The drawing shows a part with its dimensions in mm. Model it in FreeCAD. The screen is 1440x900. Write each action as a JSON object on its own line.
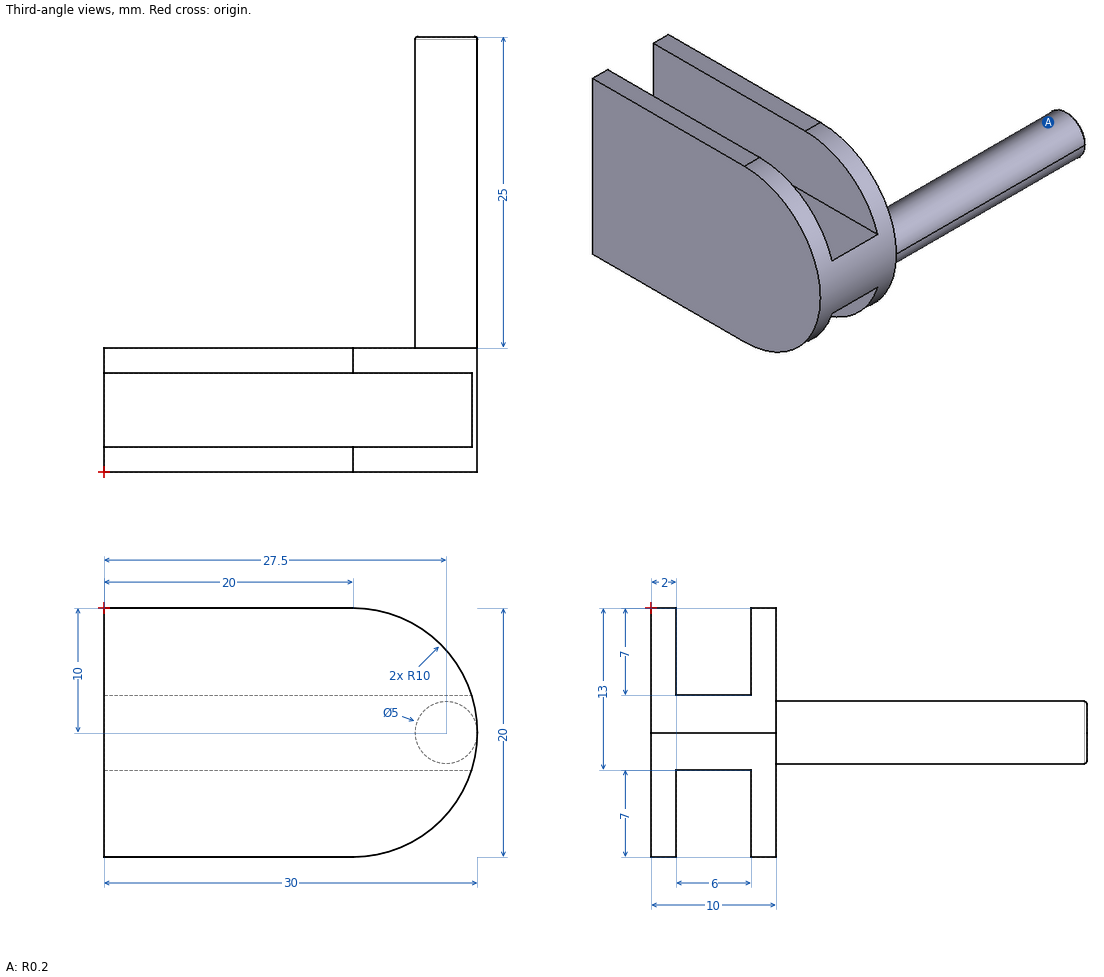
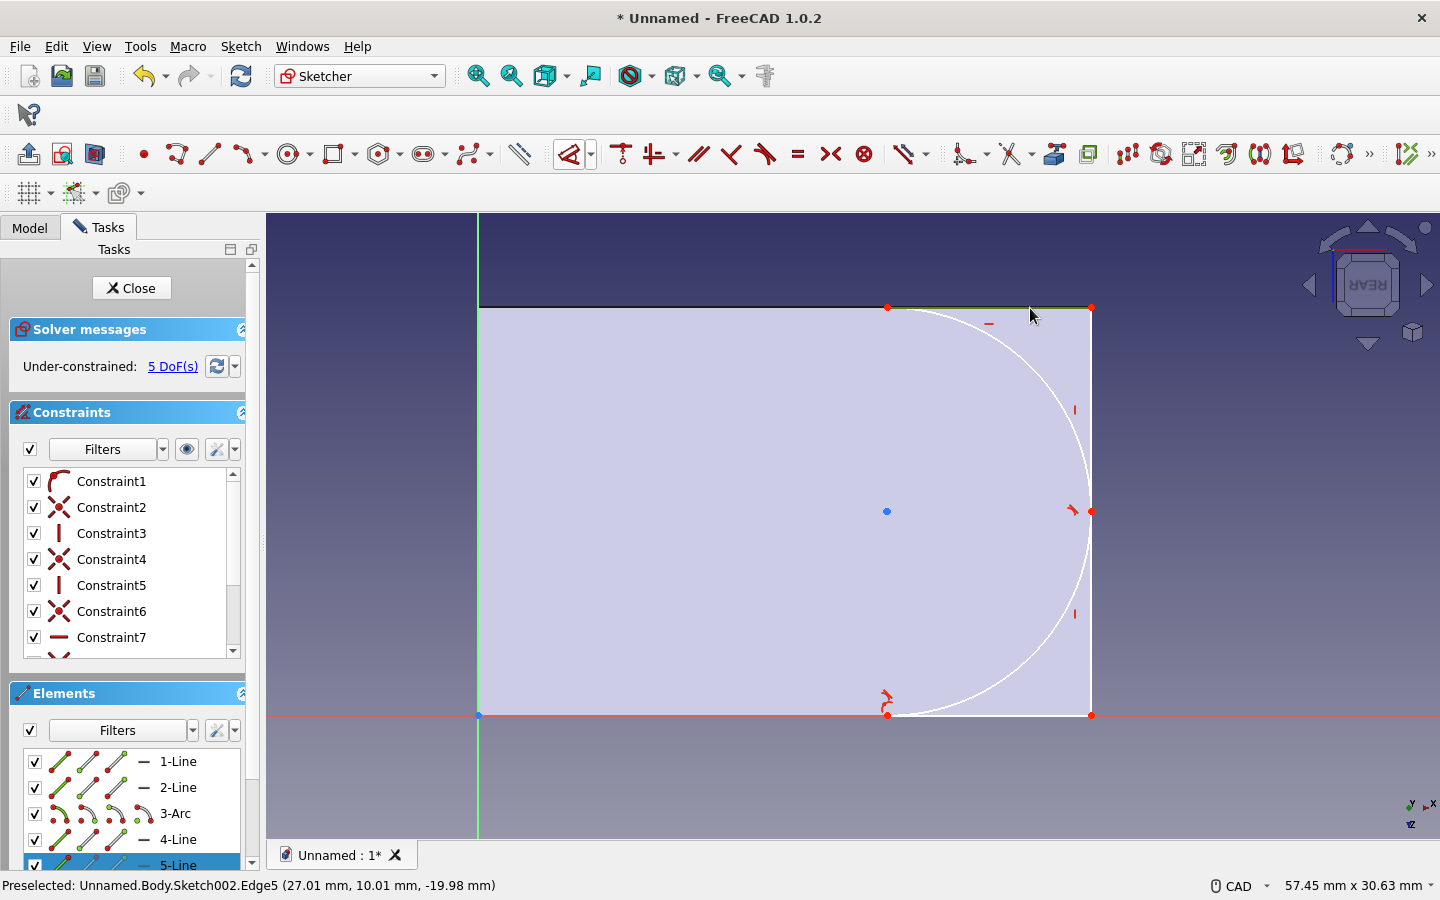
{"action": "left_click", "coordinate": [1069, 419]}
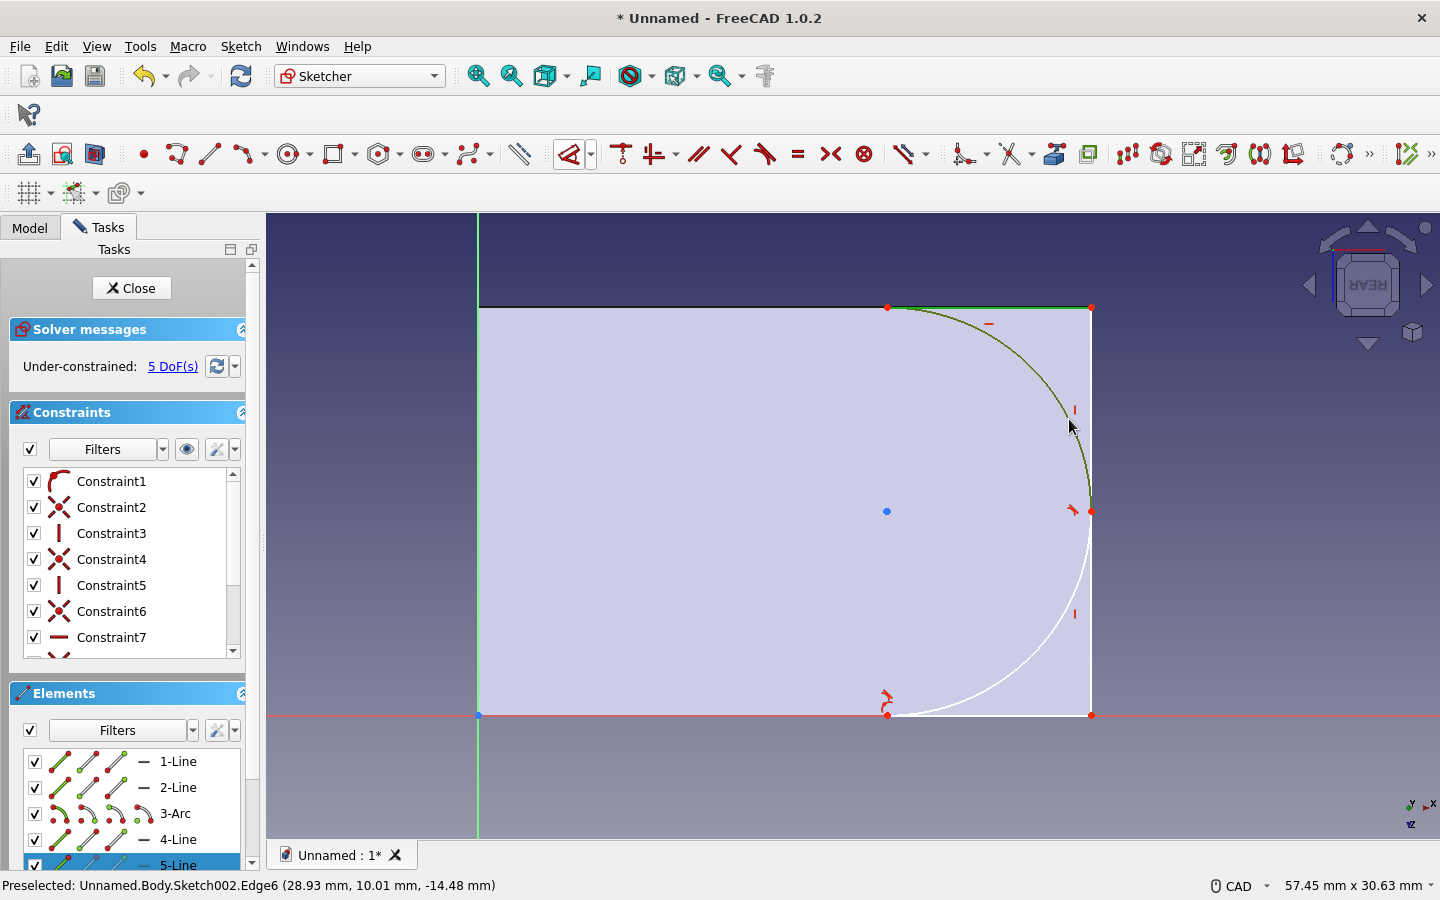
{"action": "left_click", "coordinate": [765, 154]}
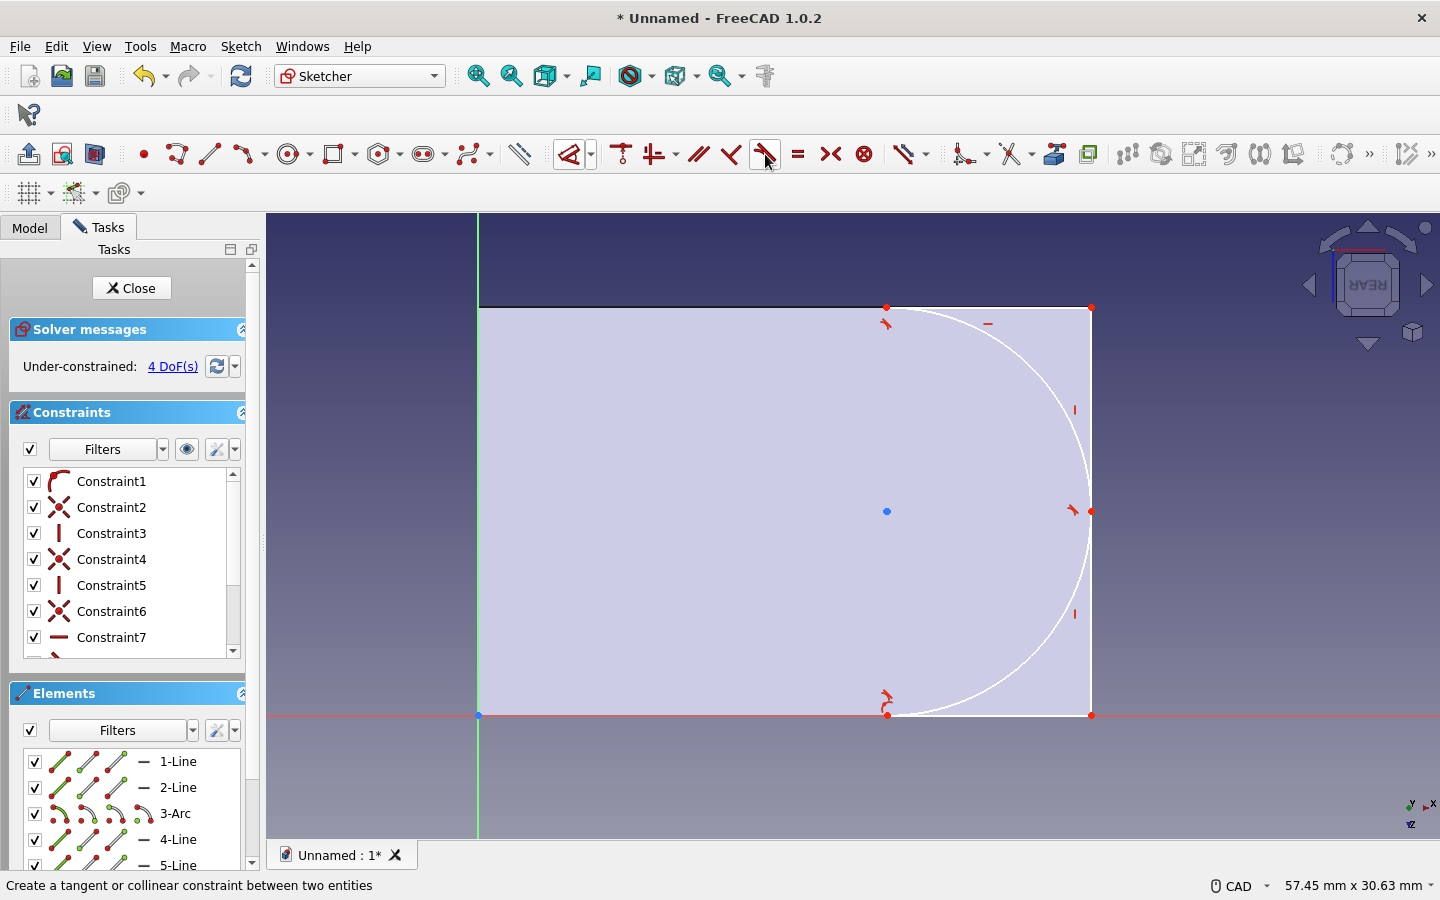
{"action": "left_click", "coordinate": [1030, 716]}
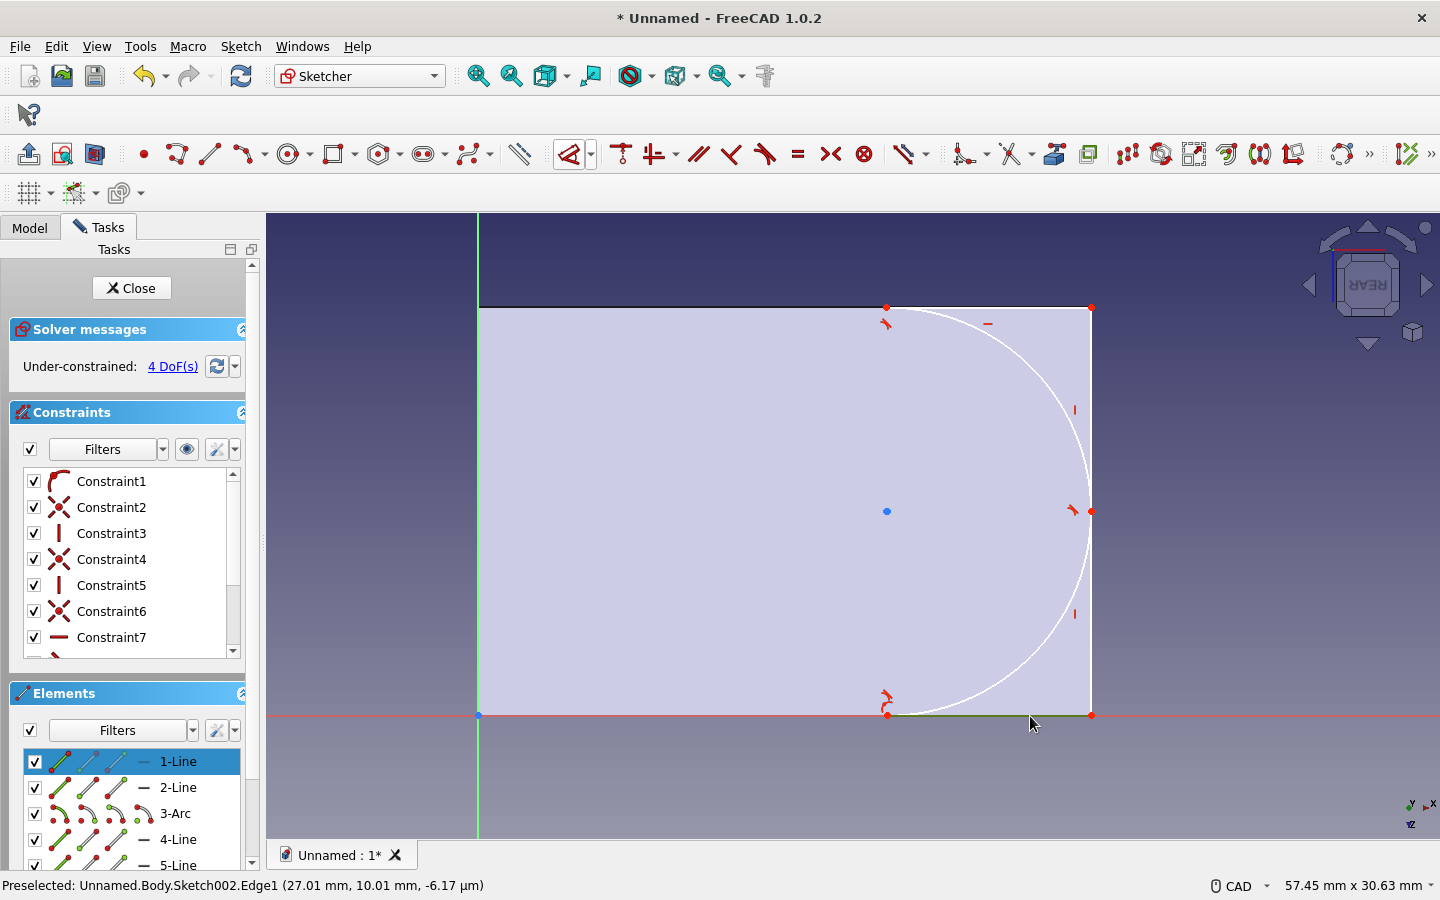
{"action": "left_click", "coordinate": [676, 154]}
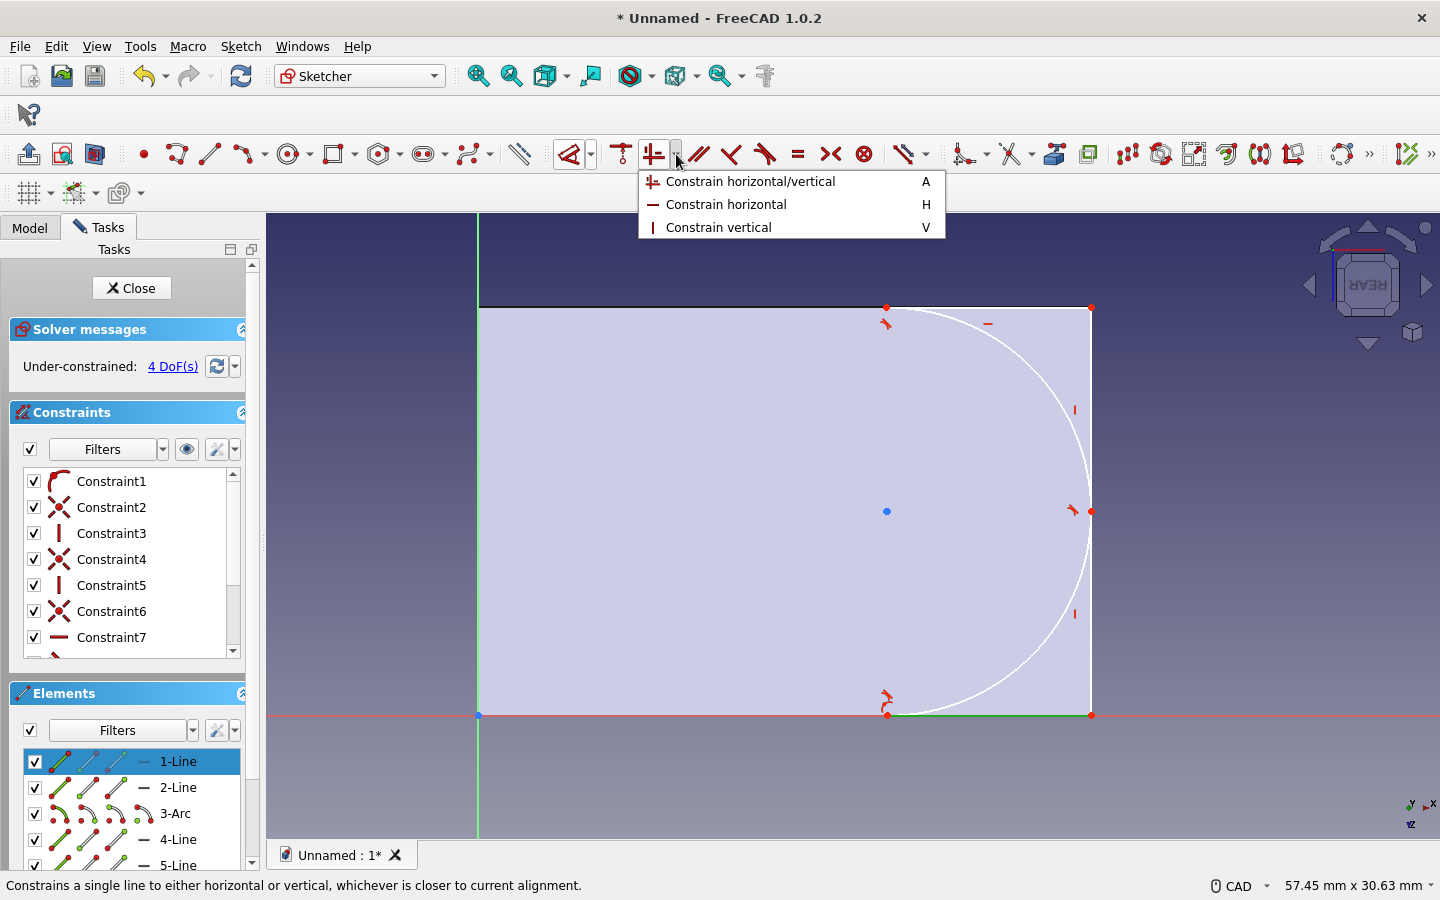
{"action": "left_click", "coordinate": [792, 204]}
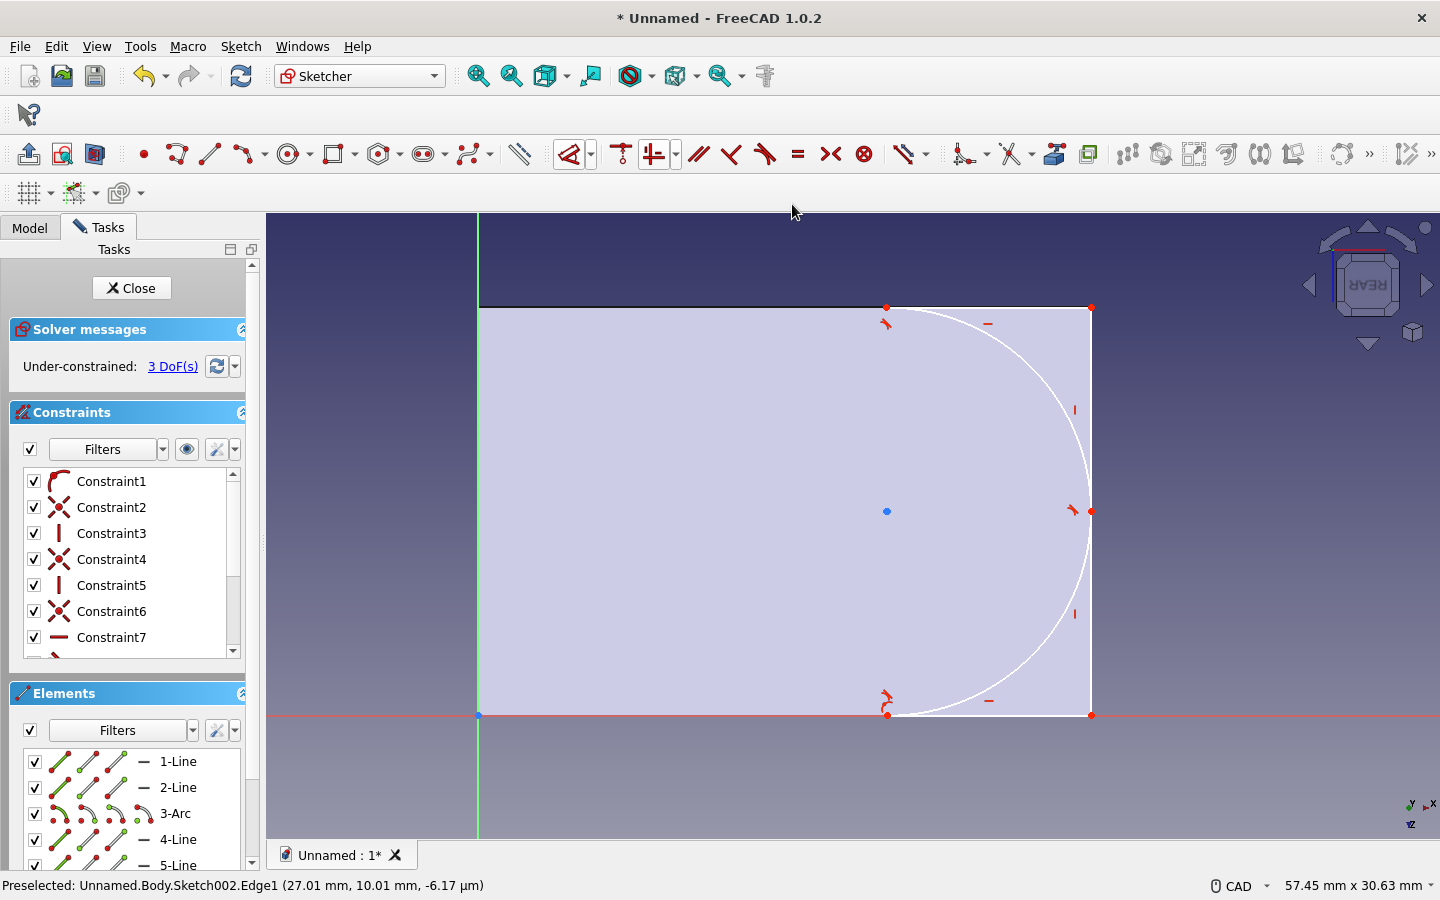
{"action": "left_click", "coordinate": [980, 694]}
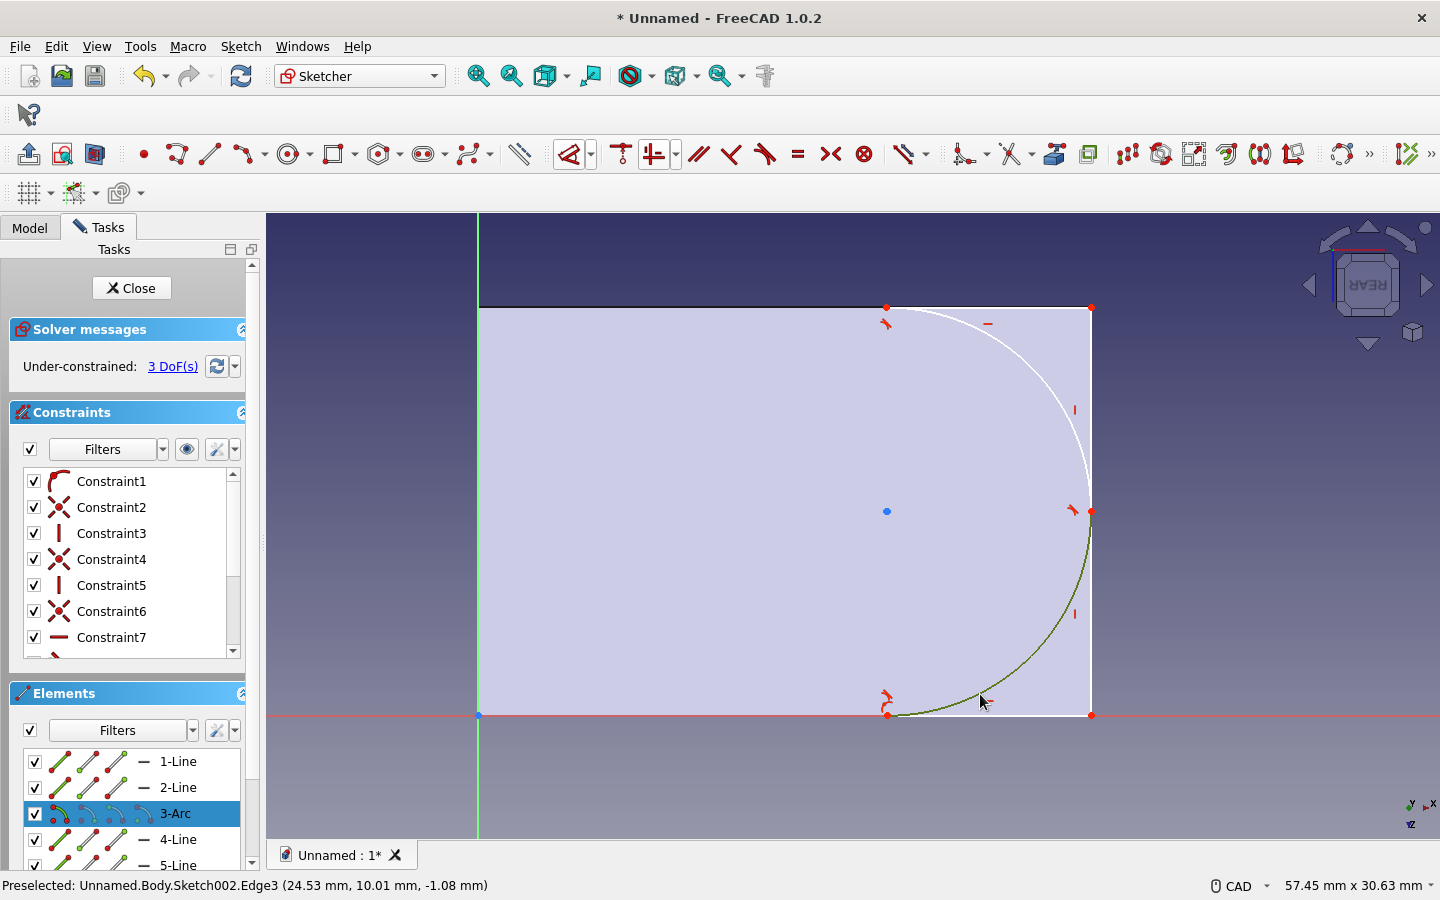
{"action": "left_click", "coordinate": [1069, 419]}